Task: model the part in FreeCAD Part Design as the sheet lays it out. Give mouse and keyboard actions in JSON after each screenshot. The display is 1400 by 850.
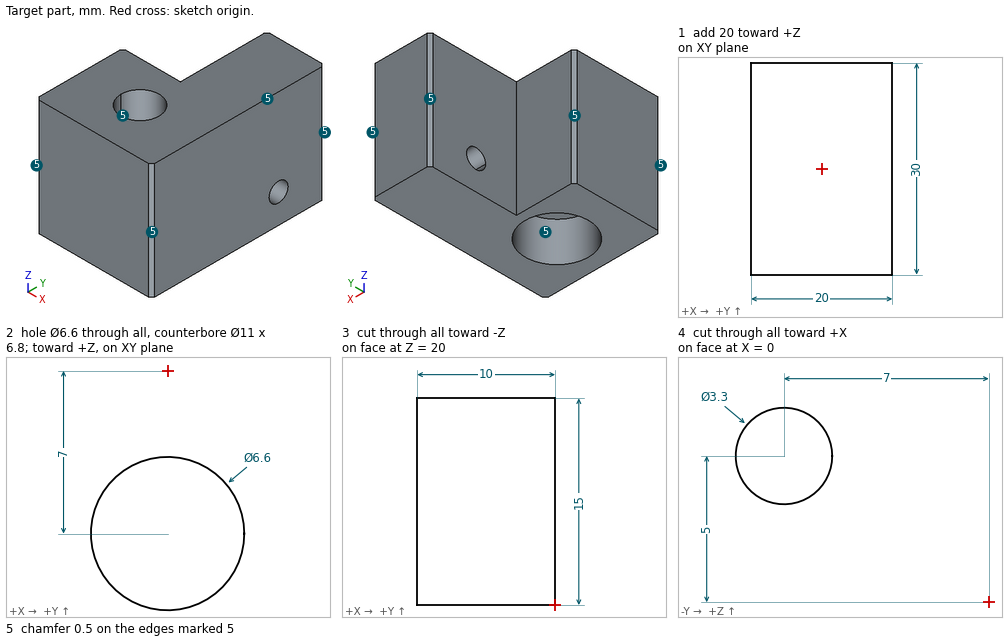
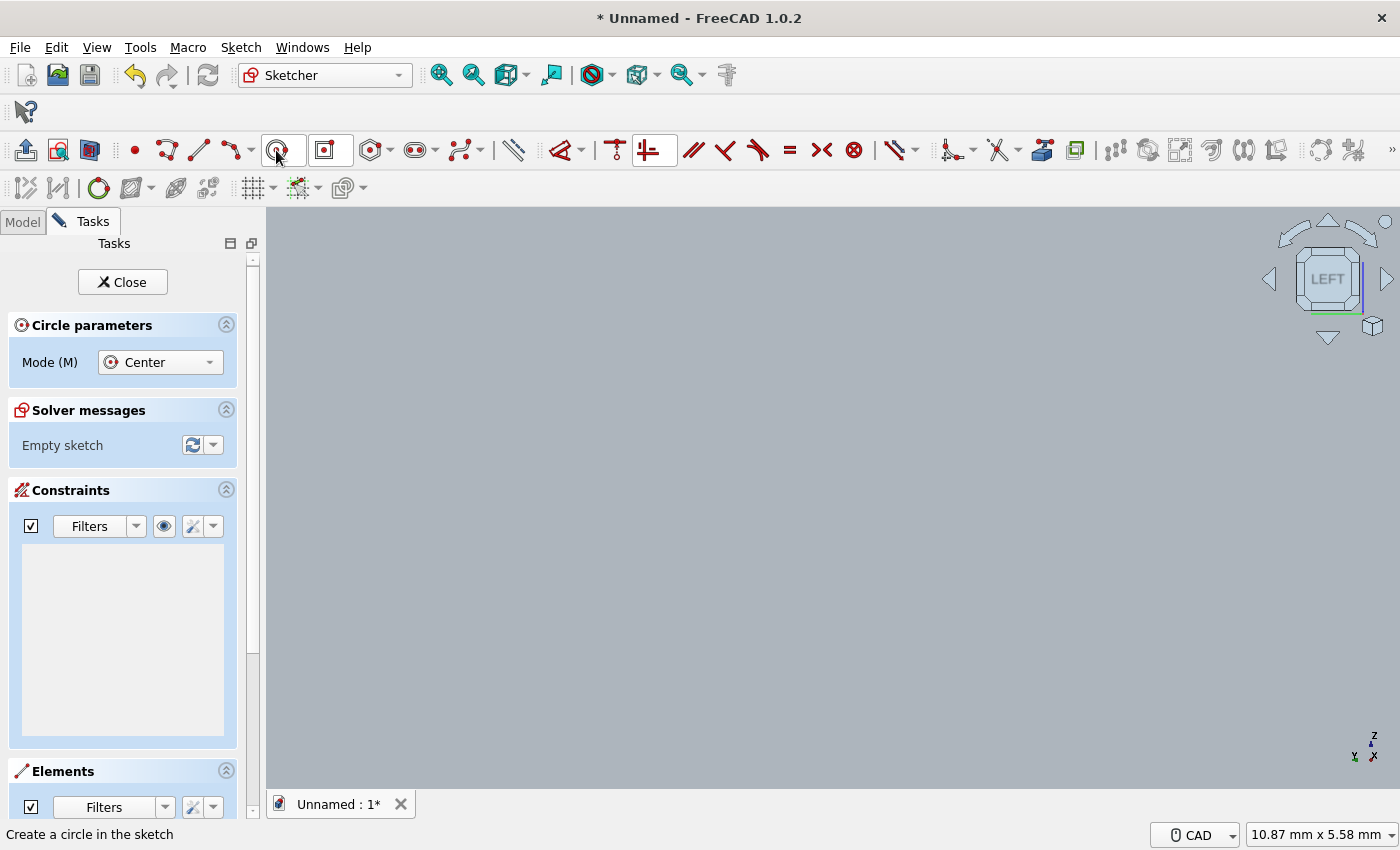
{"action": "left_click", "coordinate": [765, 491]}
{"action": "left_click", "coordinate": [886, 370]}
{"action": "key", "text": "Escape"}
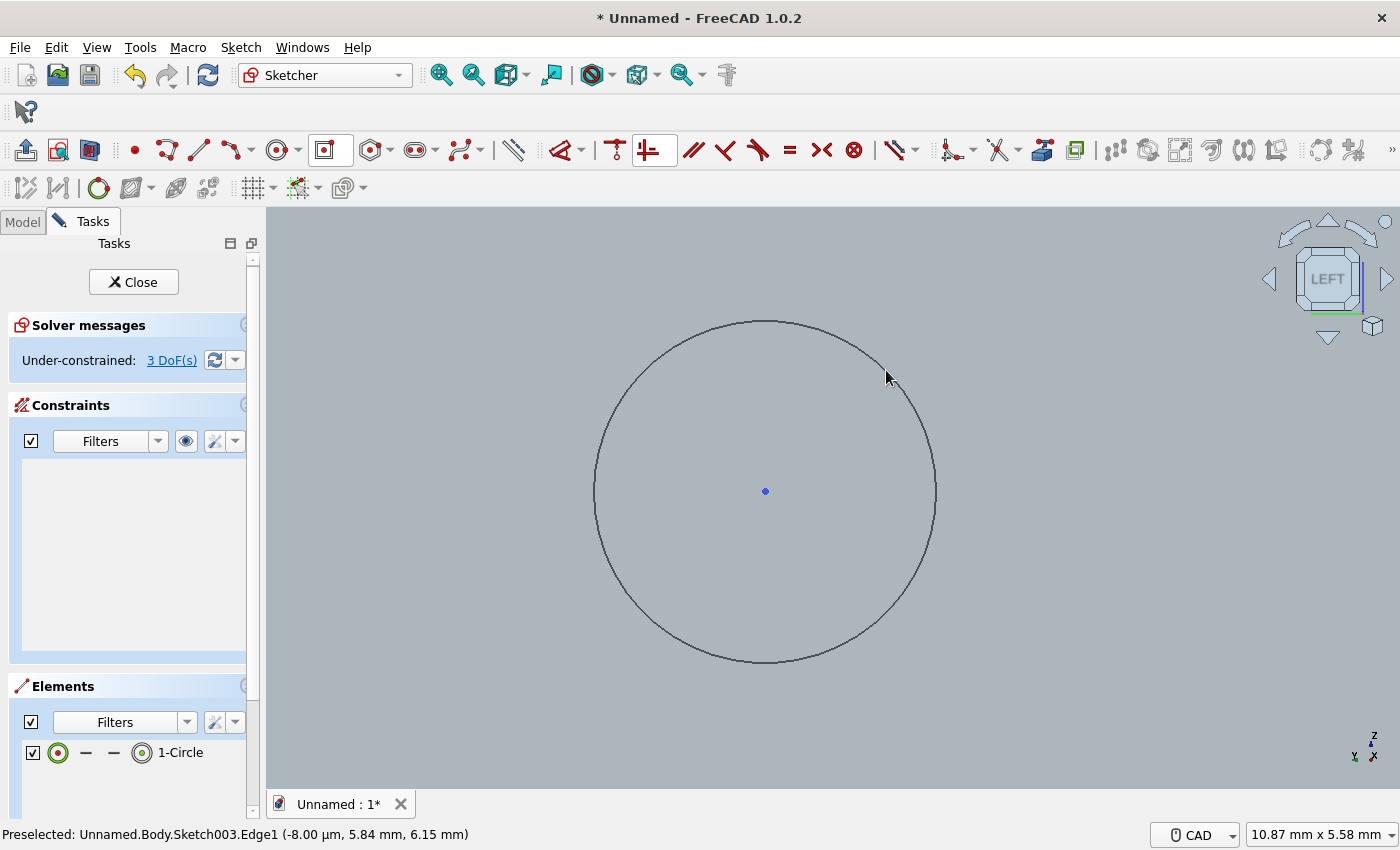
{"action": "left_click", "coordinate": [560, 150]}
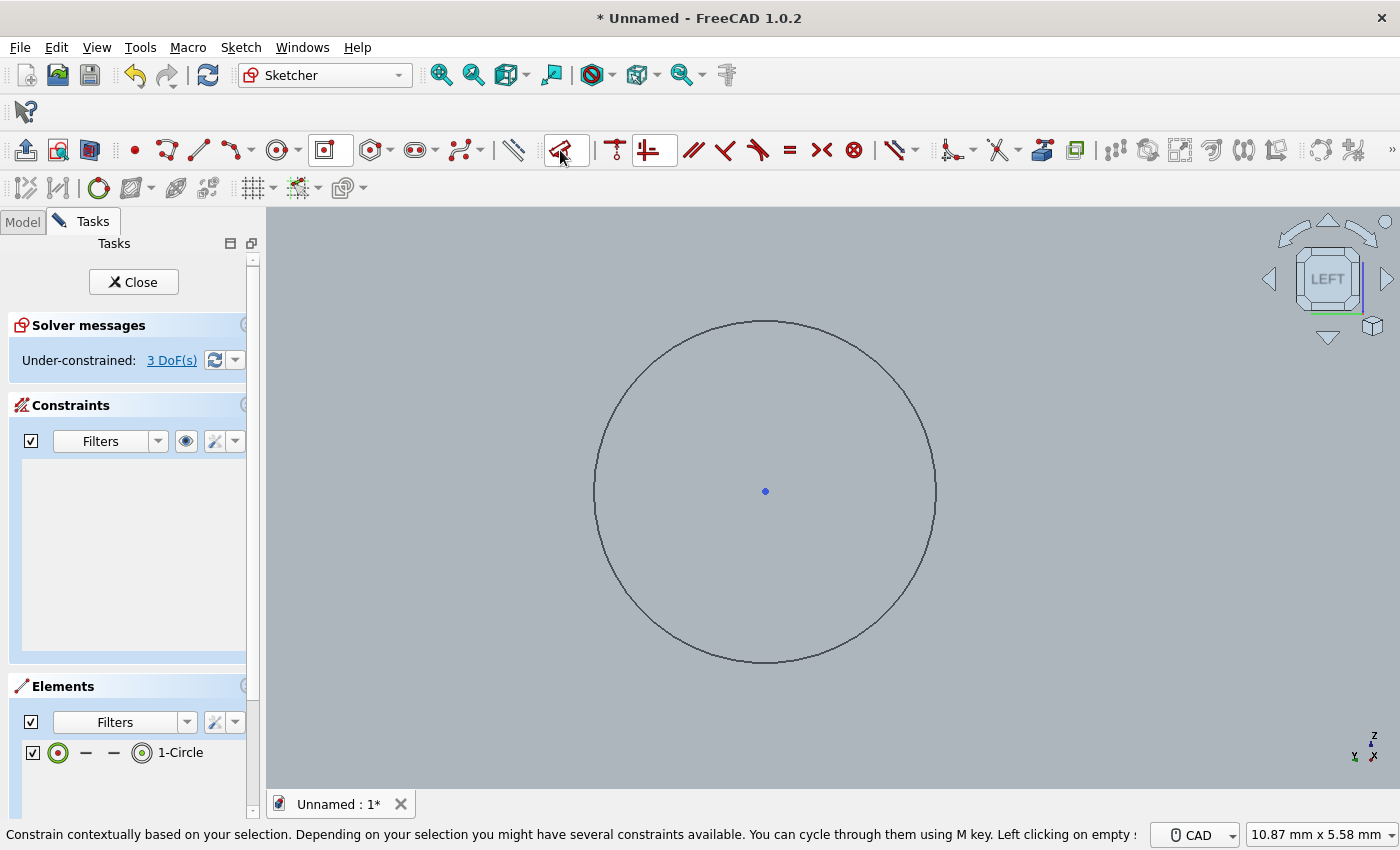
{"action": "left_click", "coordinate": [886, 371]}
{"action": "left_click", "coordinate": [909, 348]}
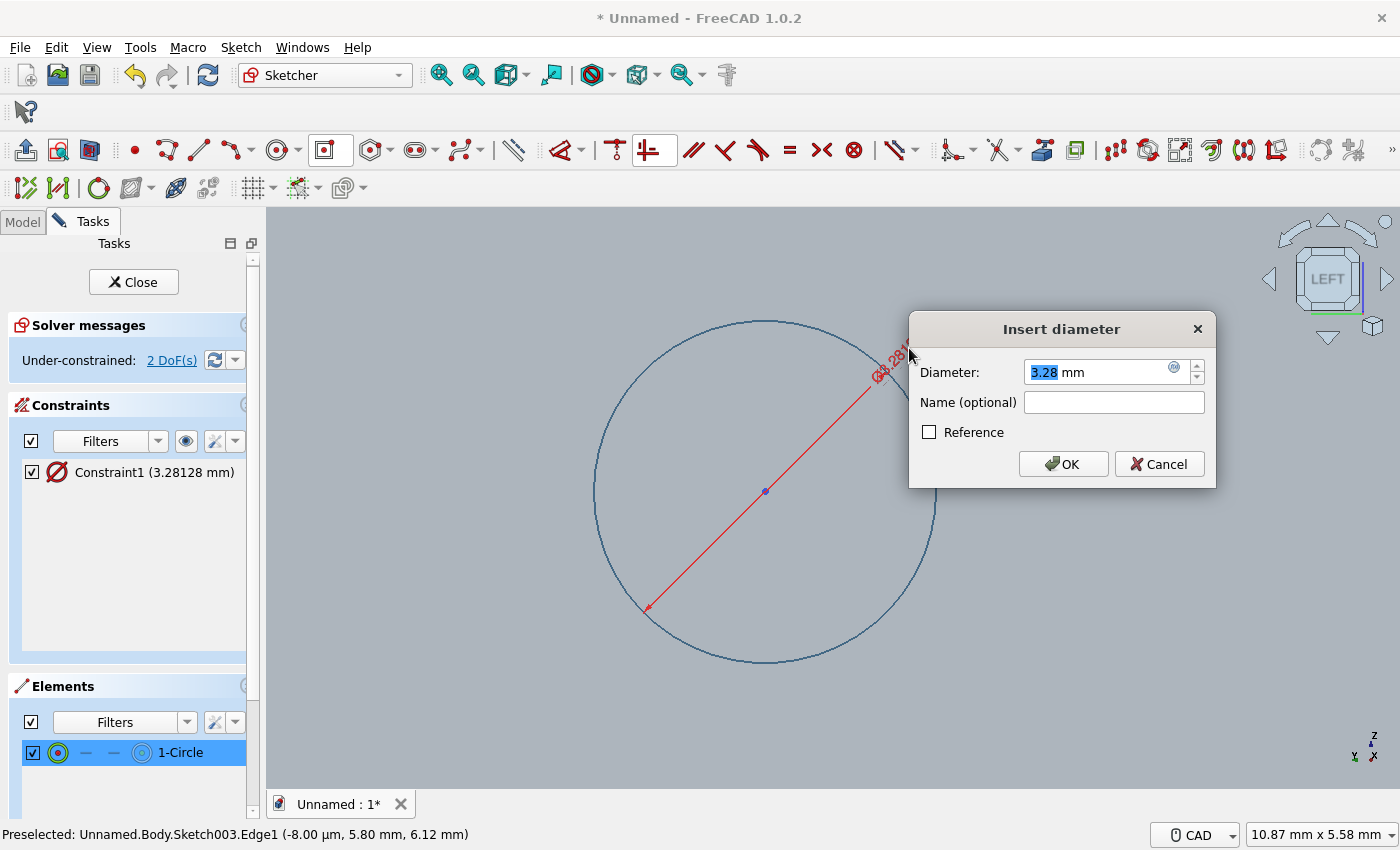
{"action": "type", "text": "3.3"}
{"action": "key", "text": "Return"}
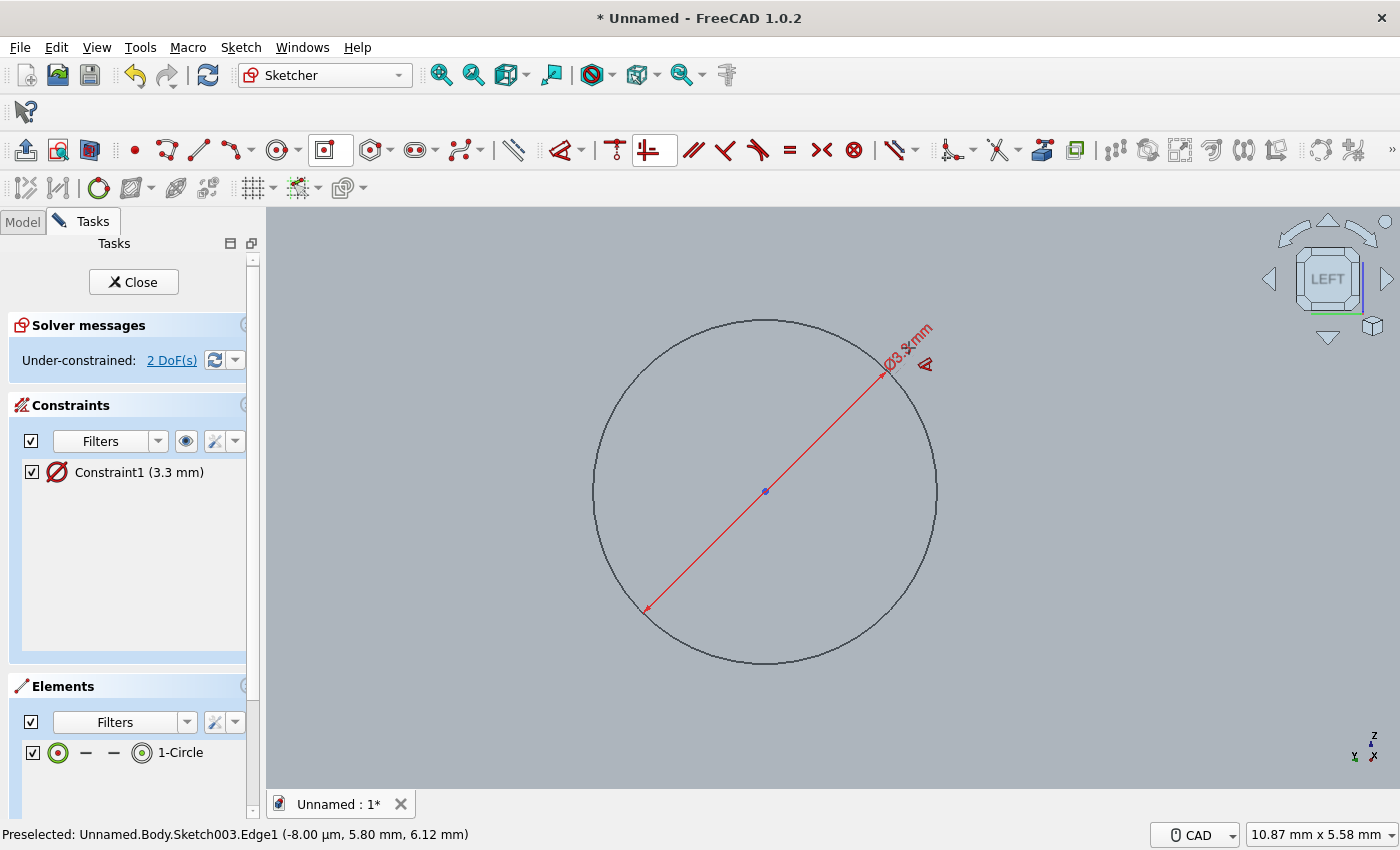
{"action": "left_click", "coordinate": [765, 492]}
{"action": "left_click", "coordinate": [1000, 458]}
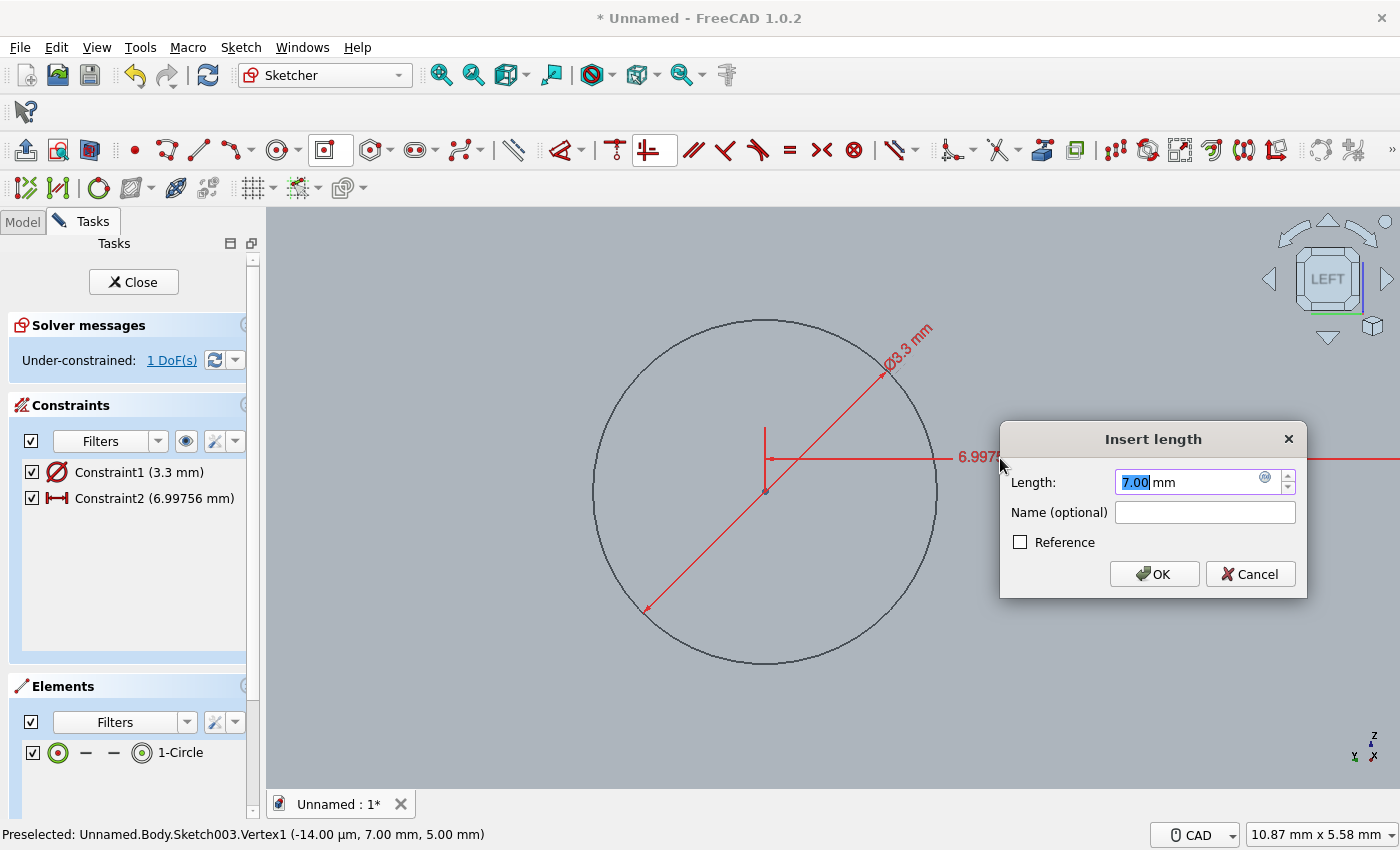
{"action": "type", "text": "7"}
{"action": "key", "text": "Return"}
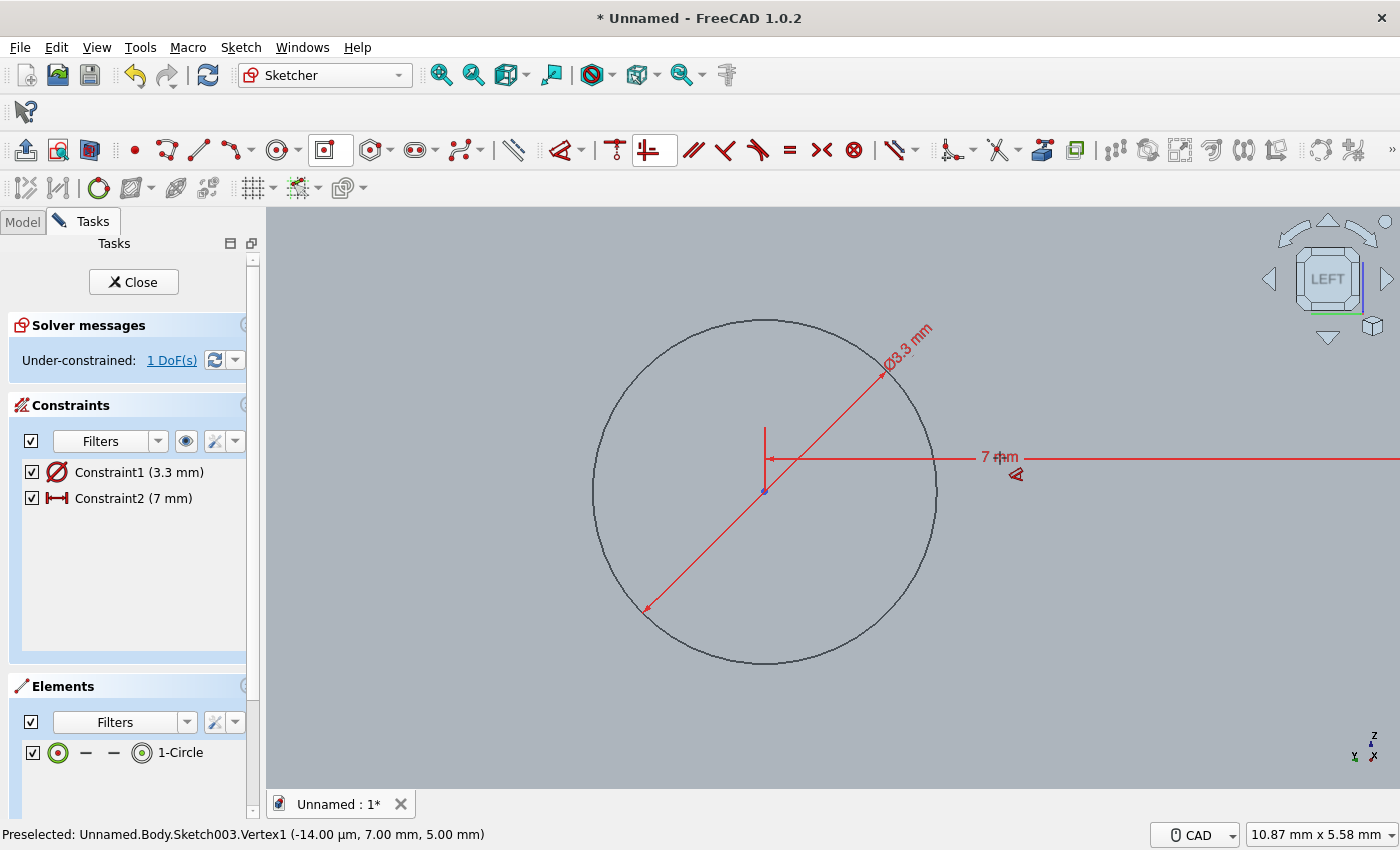
{"action": "left_click", "coordinate": [765, 492]}
{"action": "left_click", "coordinate": [731, 626]}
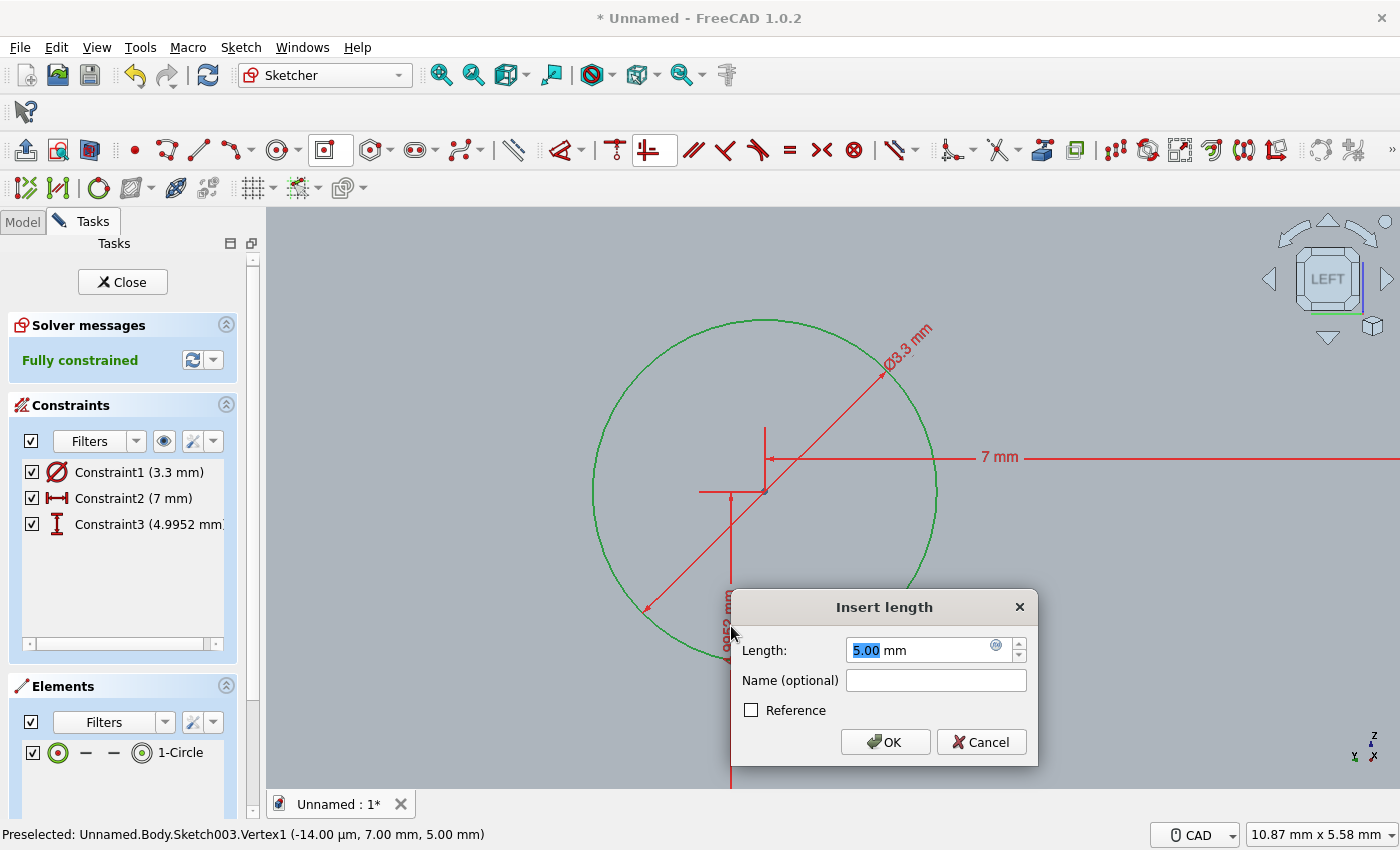
{"action": "type", "text": "5"}
{"action": "key", "text": "Return"}
{"action": "key", "text": "Escape"}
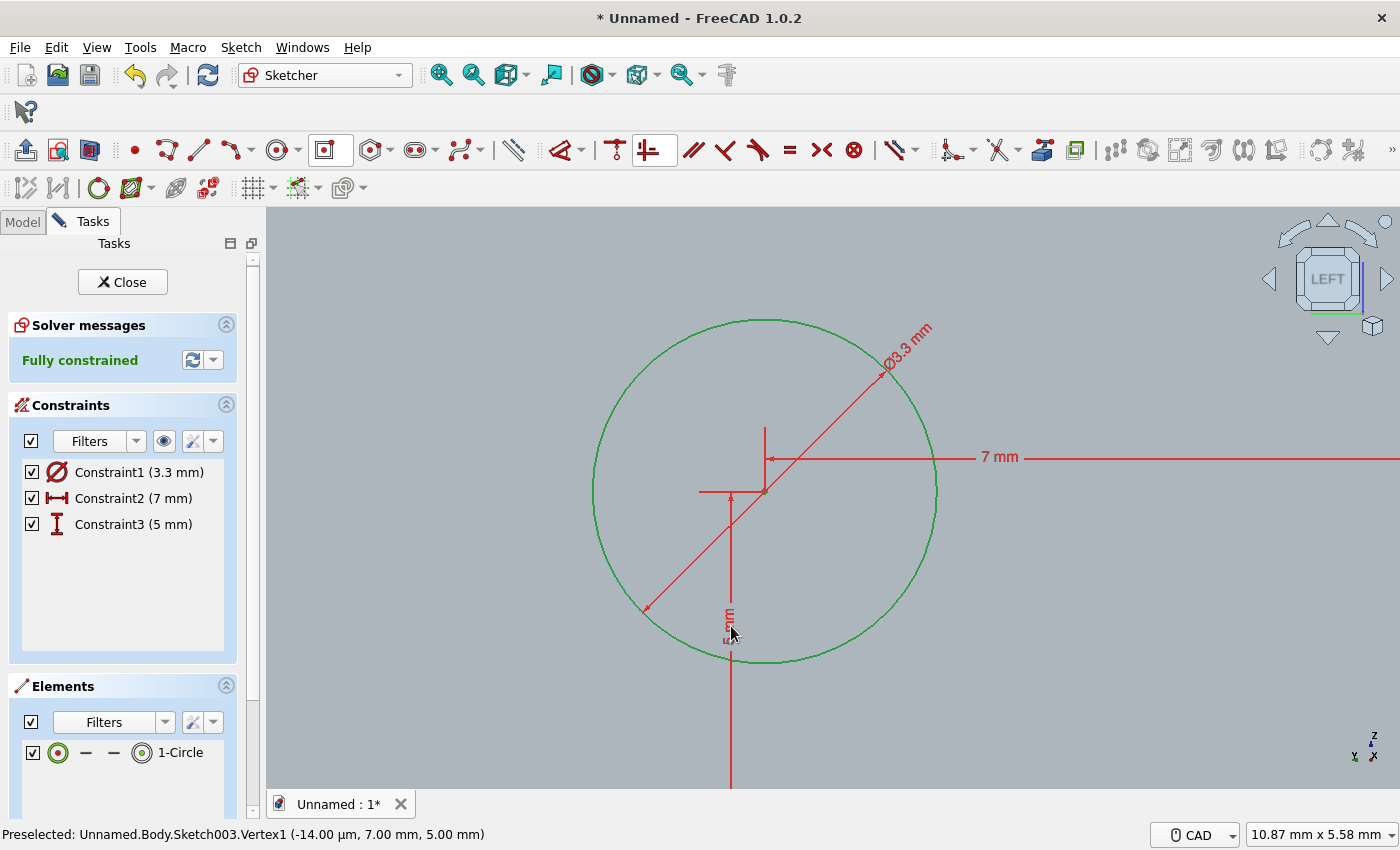
{"action": "left_click", "coordinate": [123, 282]}